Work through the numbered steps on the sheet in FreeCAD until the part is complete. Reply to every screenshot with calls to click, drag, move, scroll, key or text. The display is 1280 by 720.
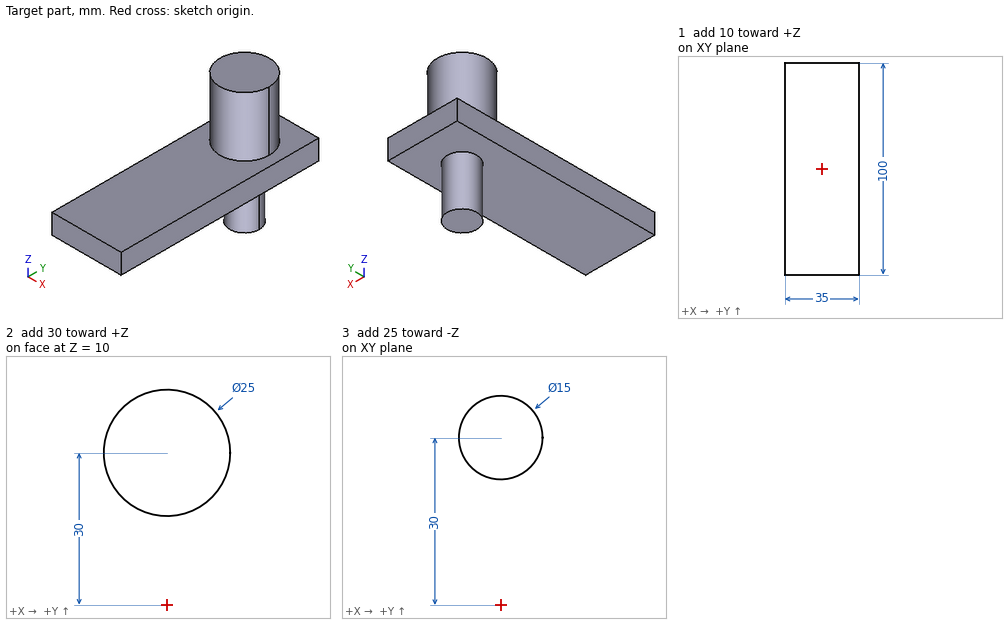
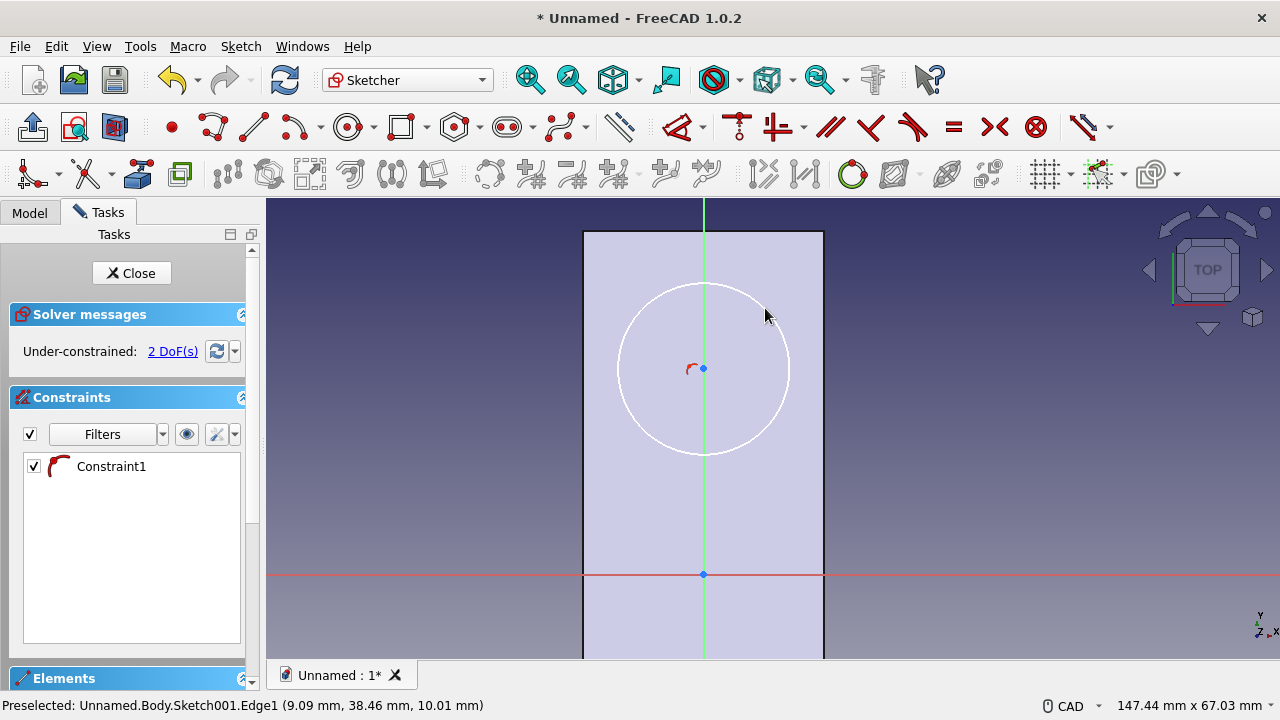
click(676, 128)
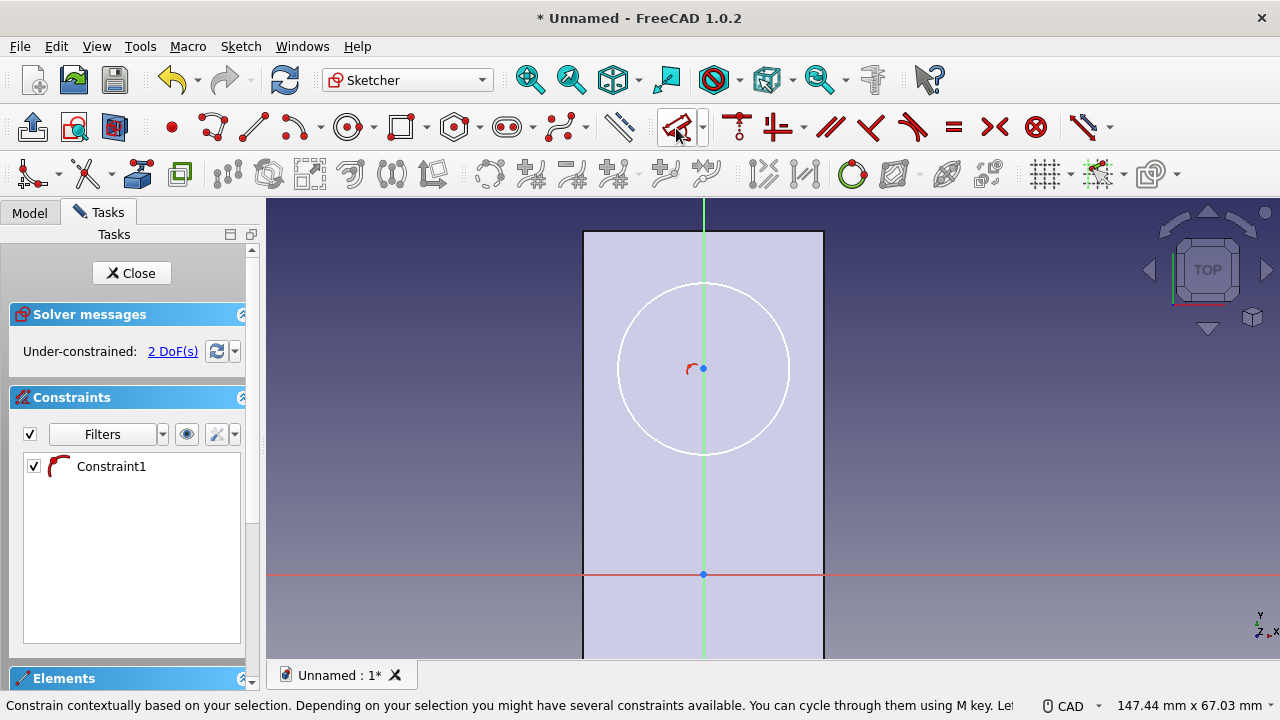
click(764, 308)
click(786, 285)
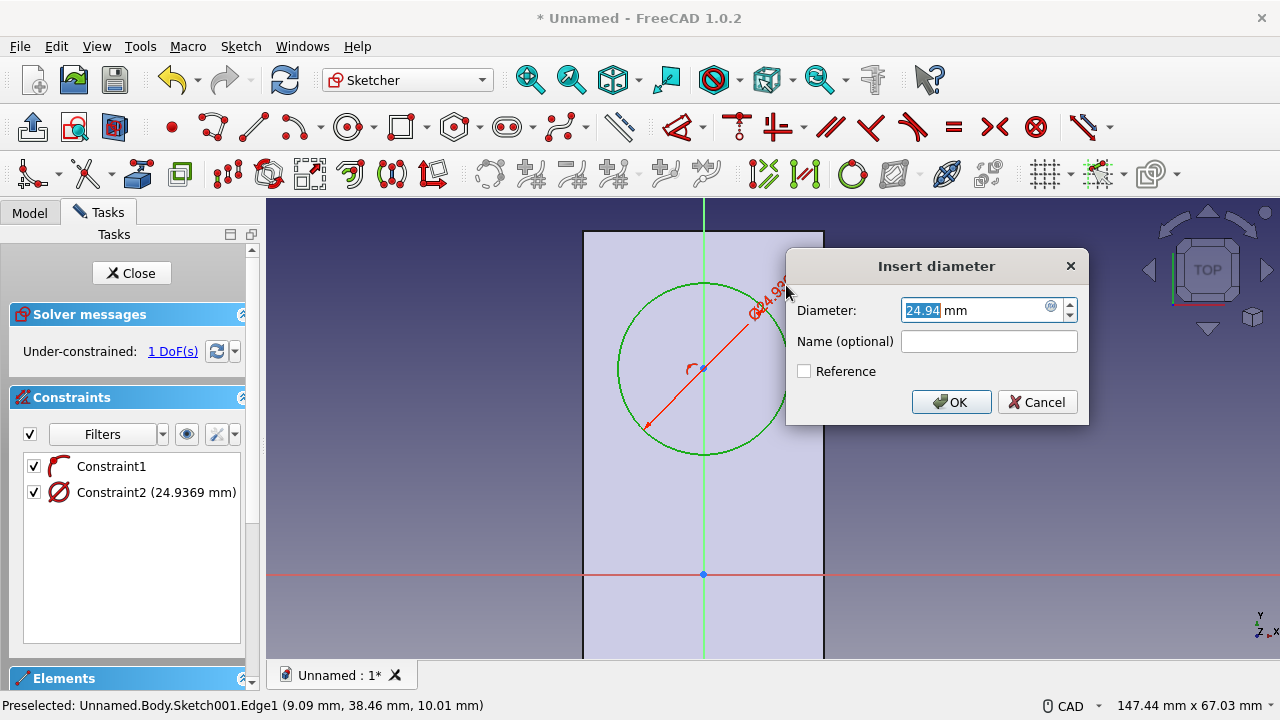
text(25)
key(Return)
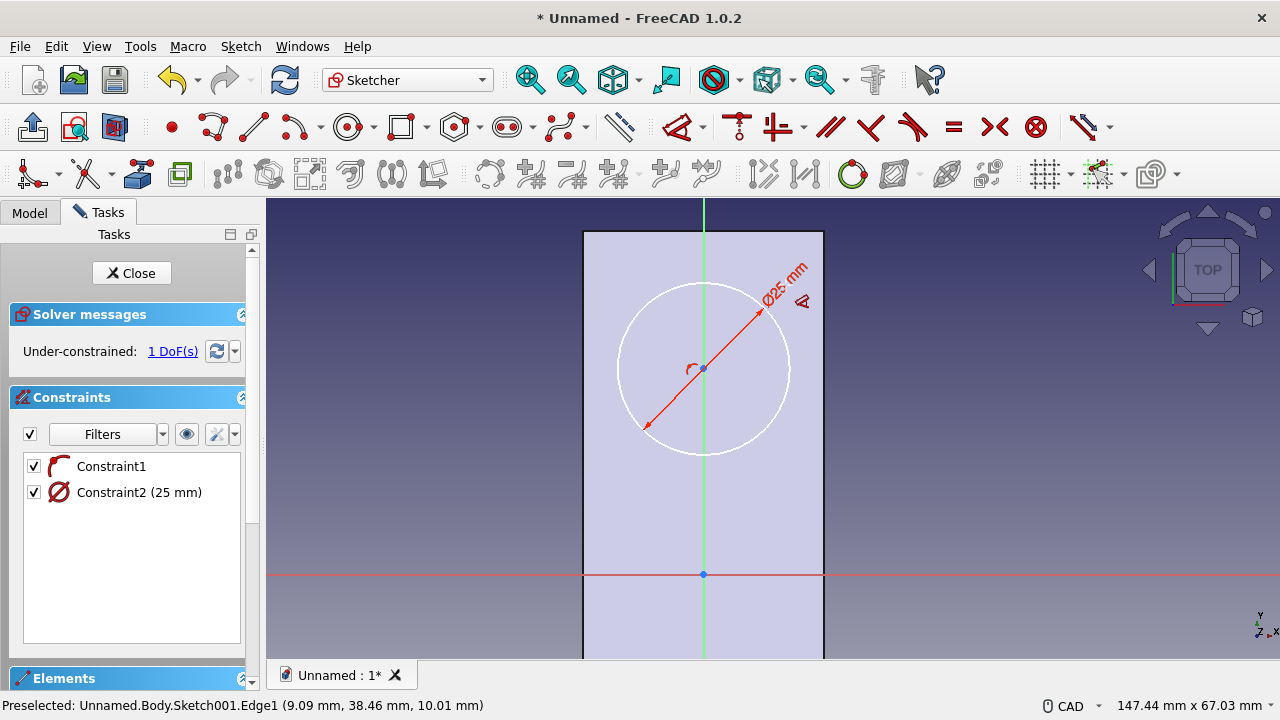
click(704, 369)
click(738, 472)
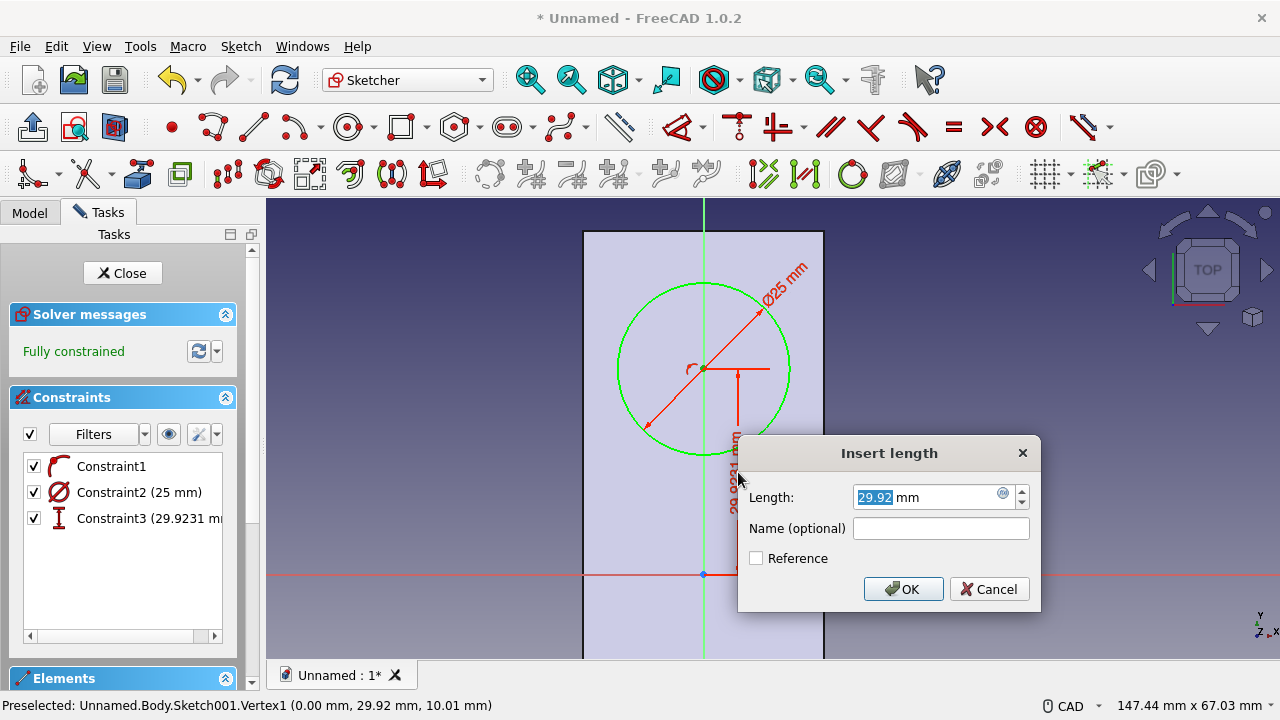
text(30)
key(Return)
key(Escape)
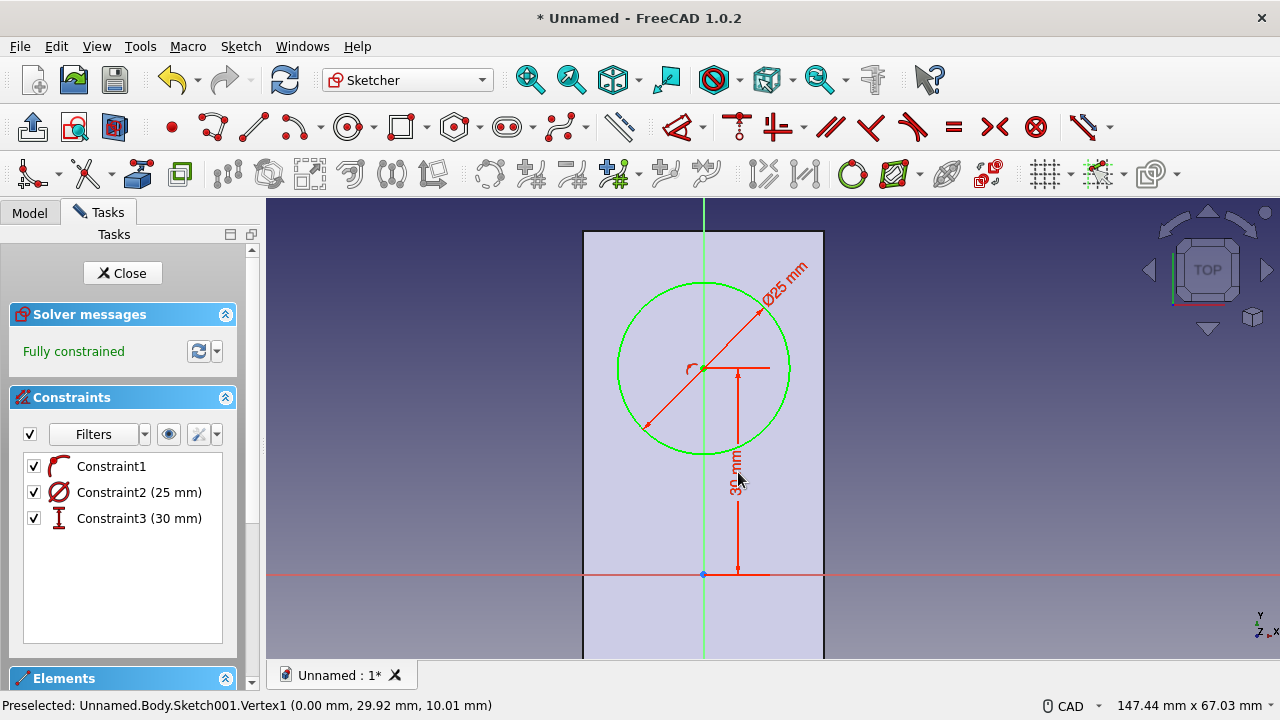
click(123, 273)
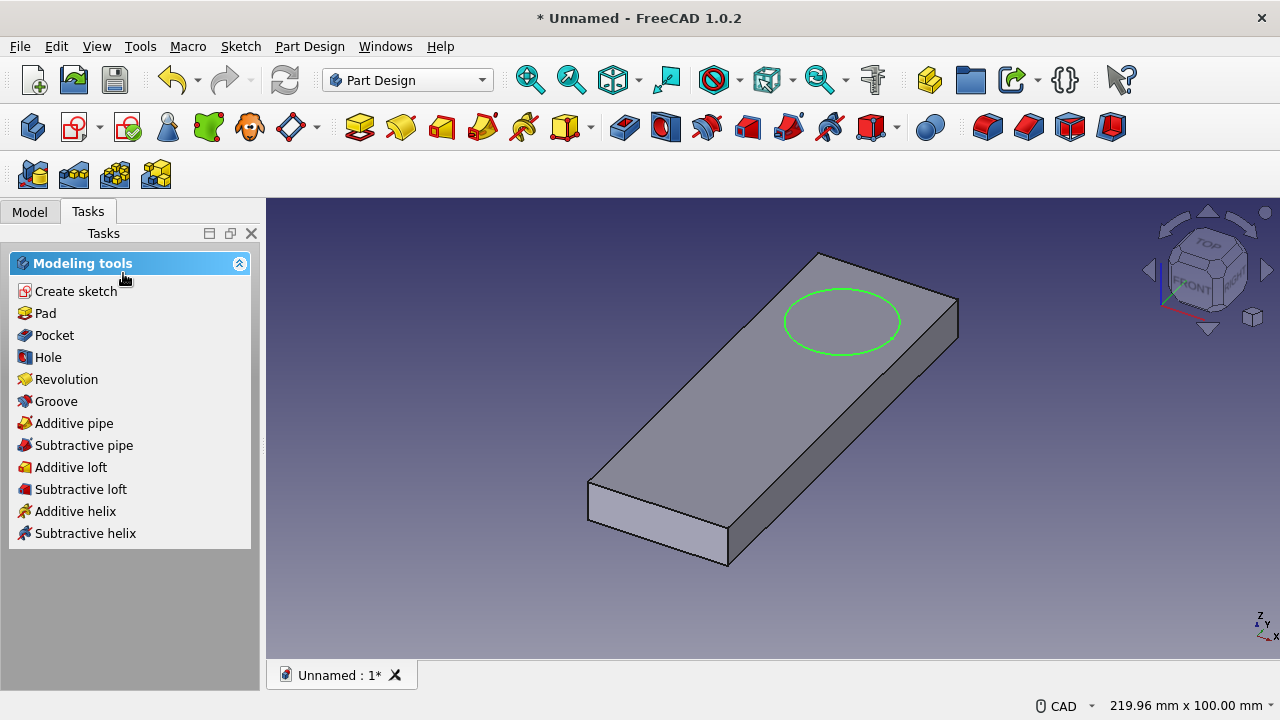
click(360, 128)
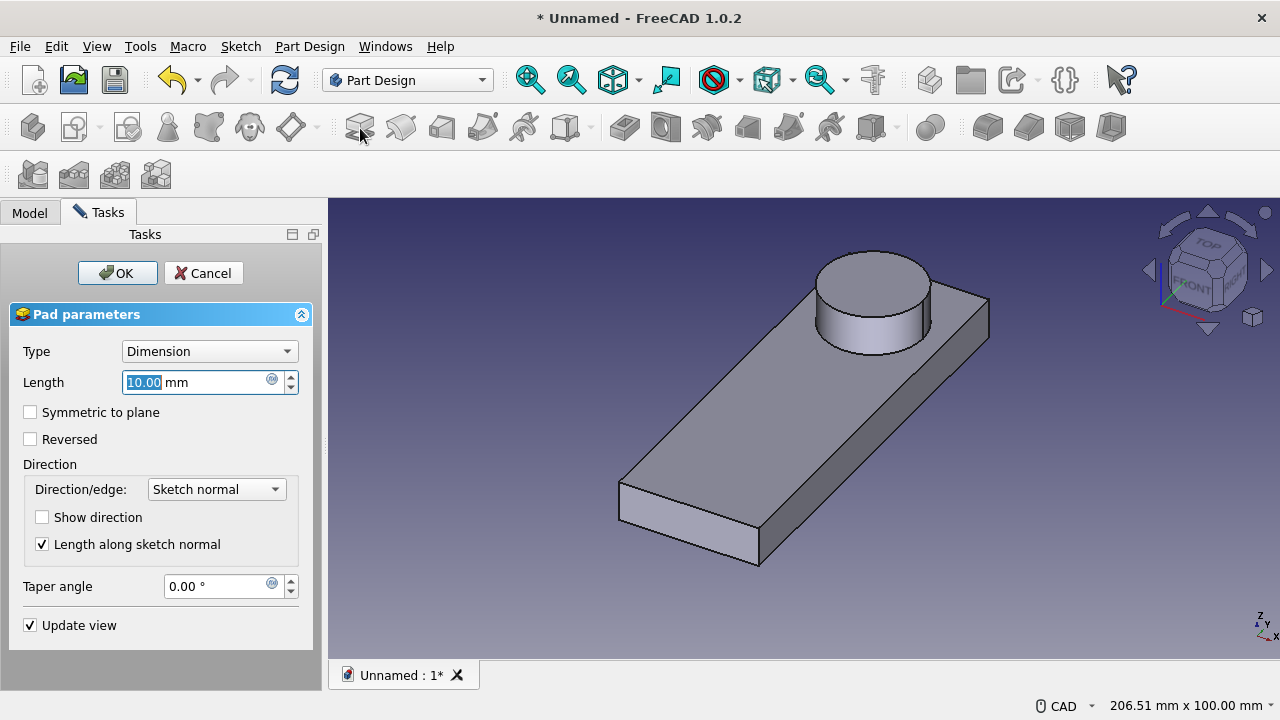
text(30)
key(Tab)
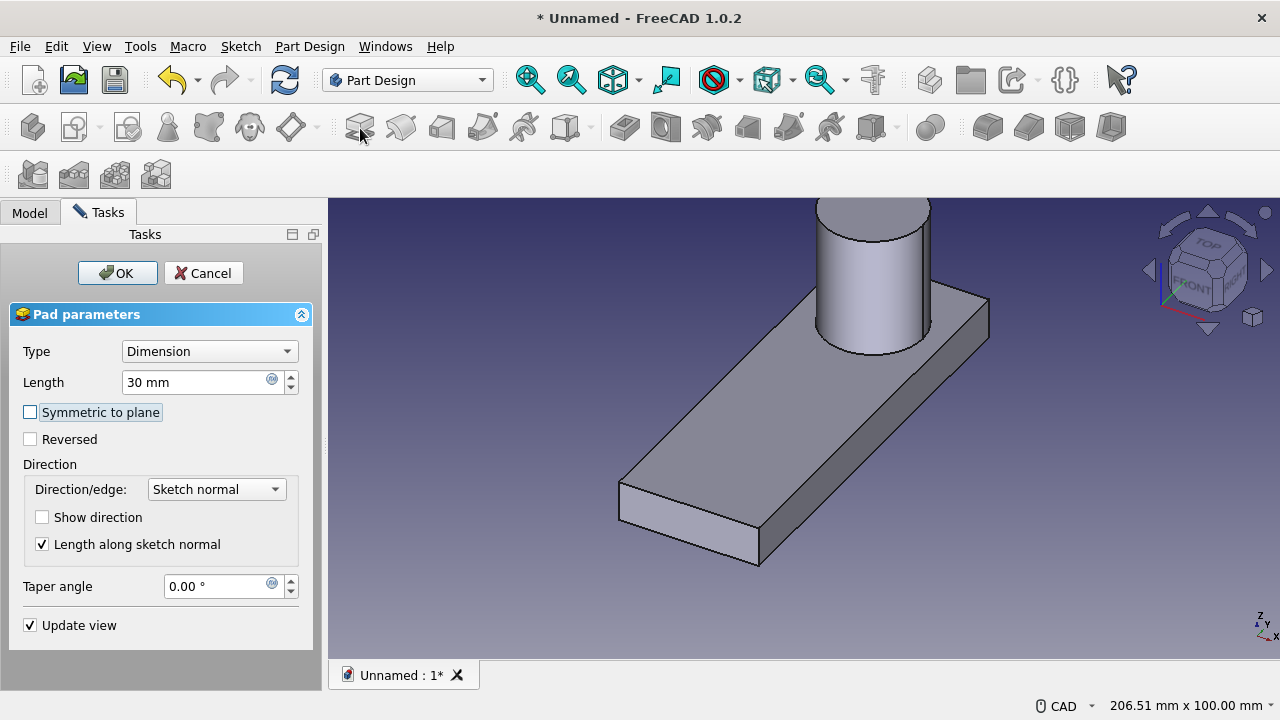
click(118, 273)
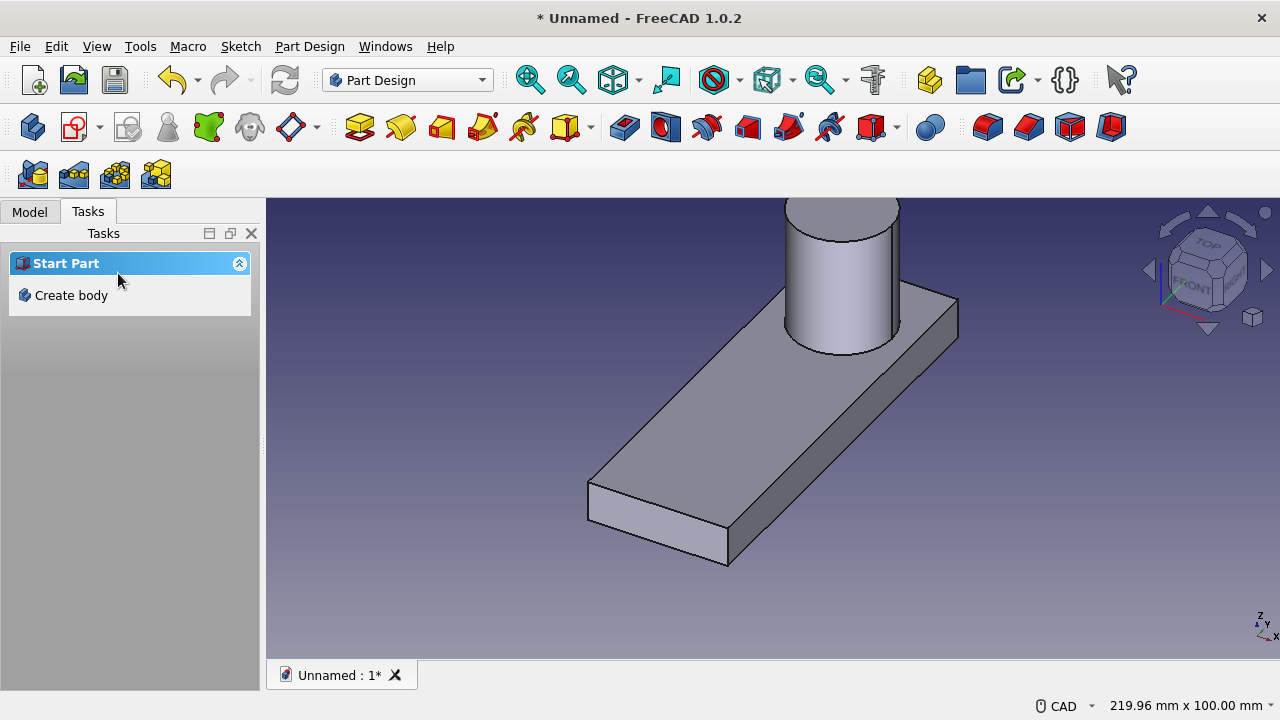
click(531, 80)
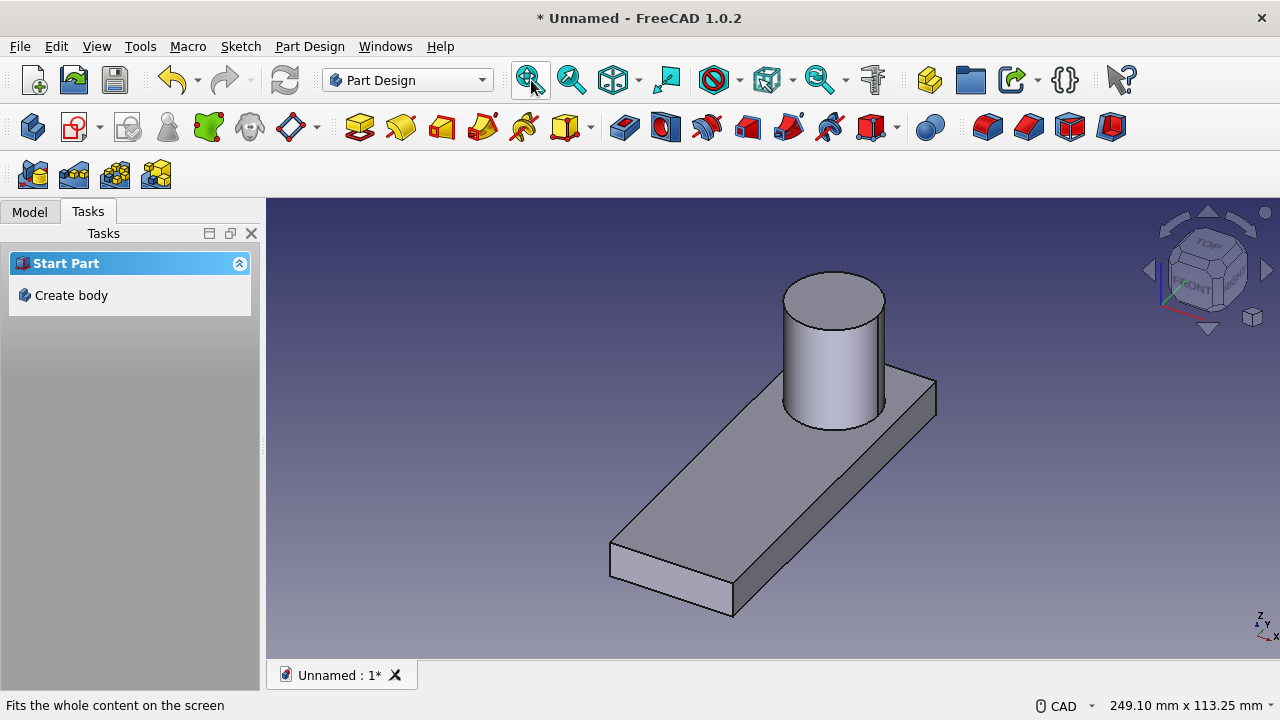
click(74, 128)